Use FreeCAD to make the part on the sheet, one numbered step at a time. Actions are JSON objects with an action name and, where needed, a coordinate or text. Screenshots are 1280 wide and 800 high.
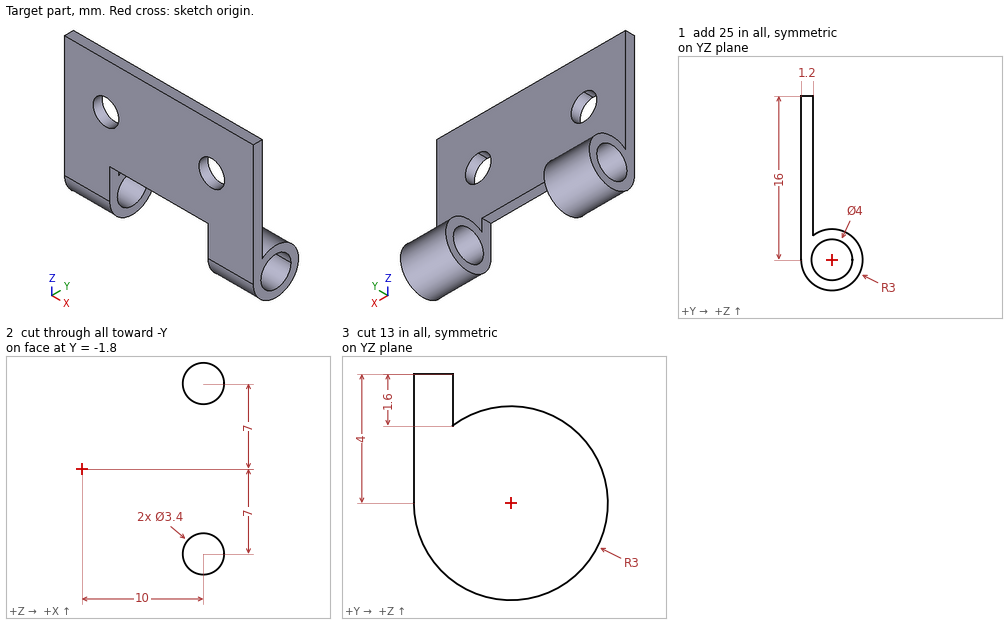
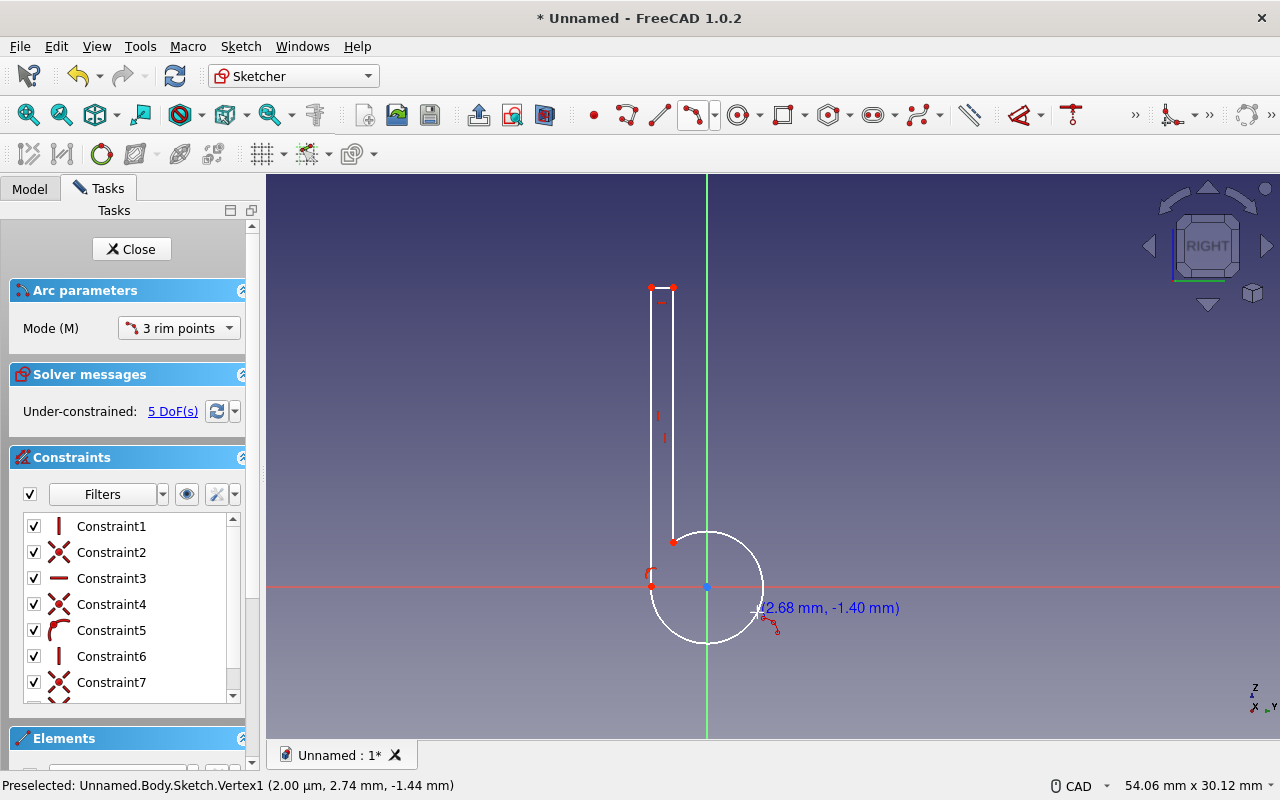
{"action": "key", "text": "g c"}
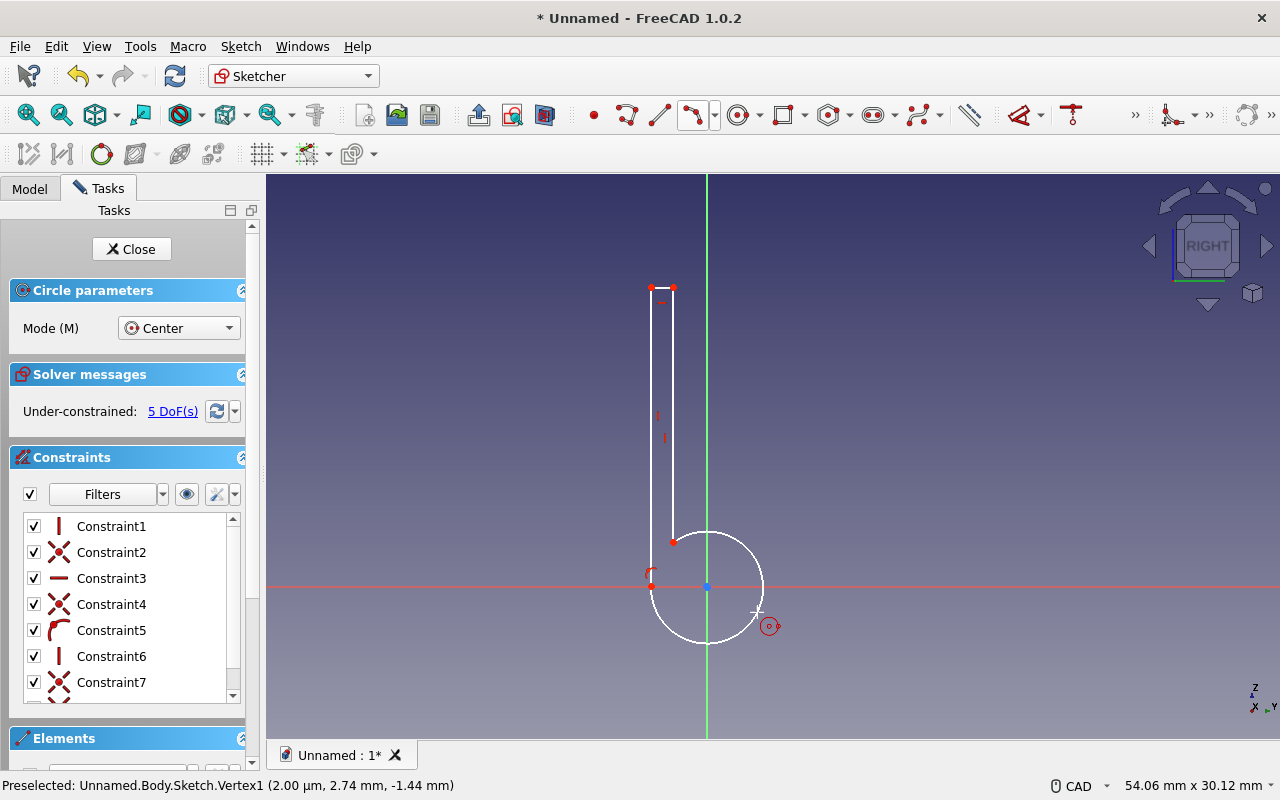
{"action": "left_click", "coordinate": [707, 587]}
{"action": "left_click", "coordinate": [733, 560]}
{"action": "key", "text": "Escape"}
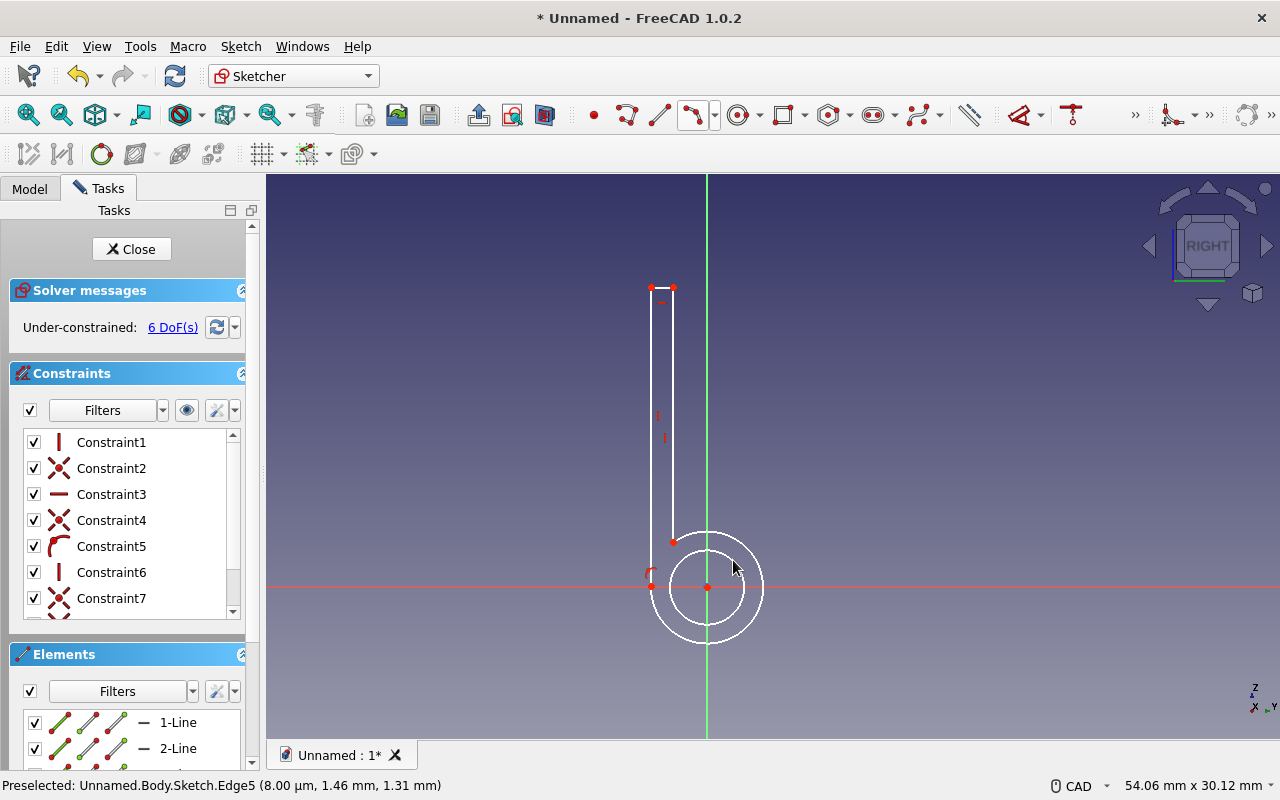
{"action": "left_click", "coordinate": [651, 378]}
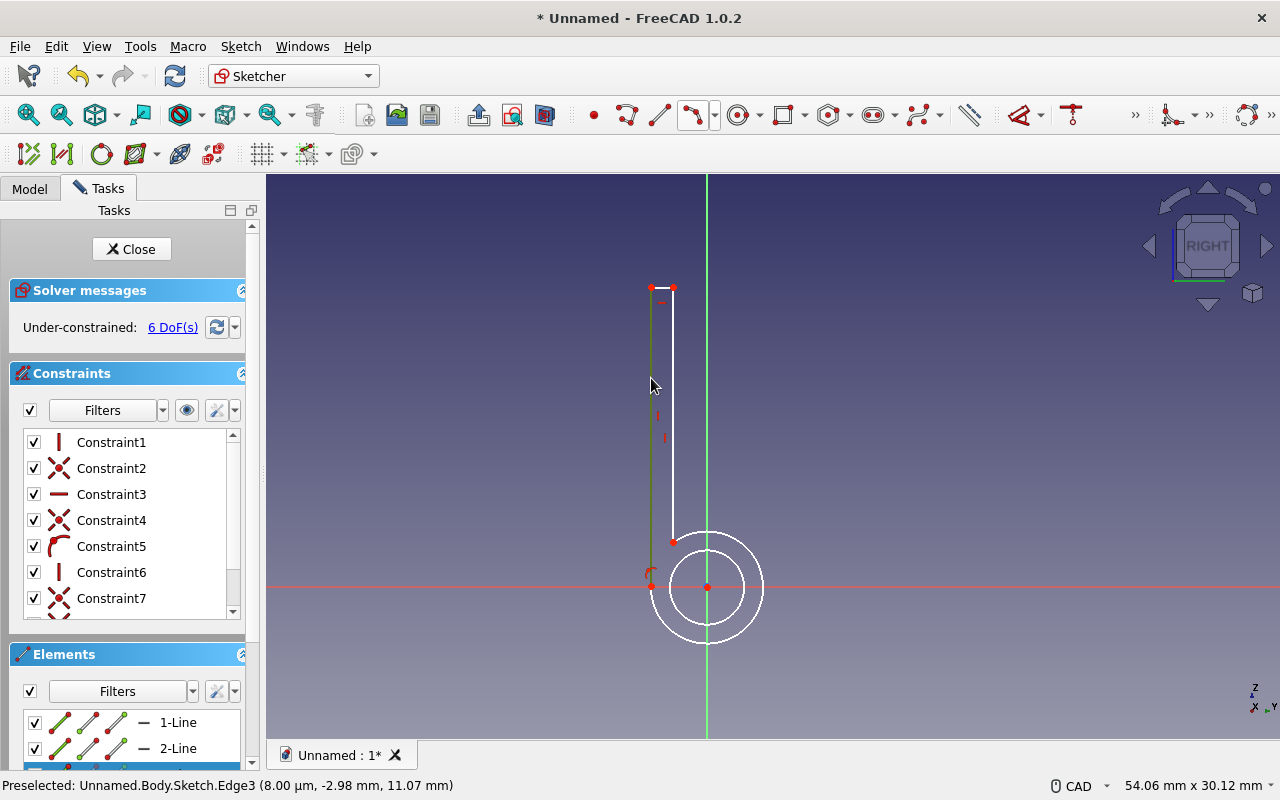
{"action": "left_click", "coordinate": [709, 644]}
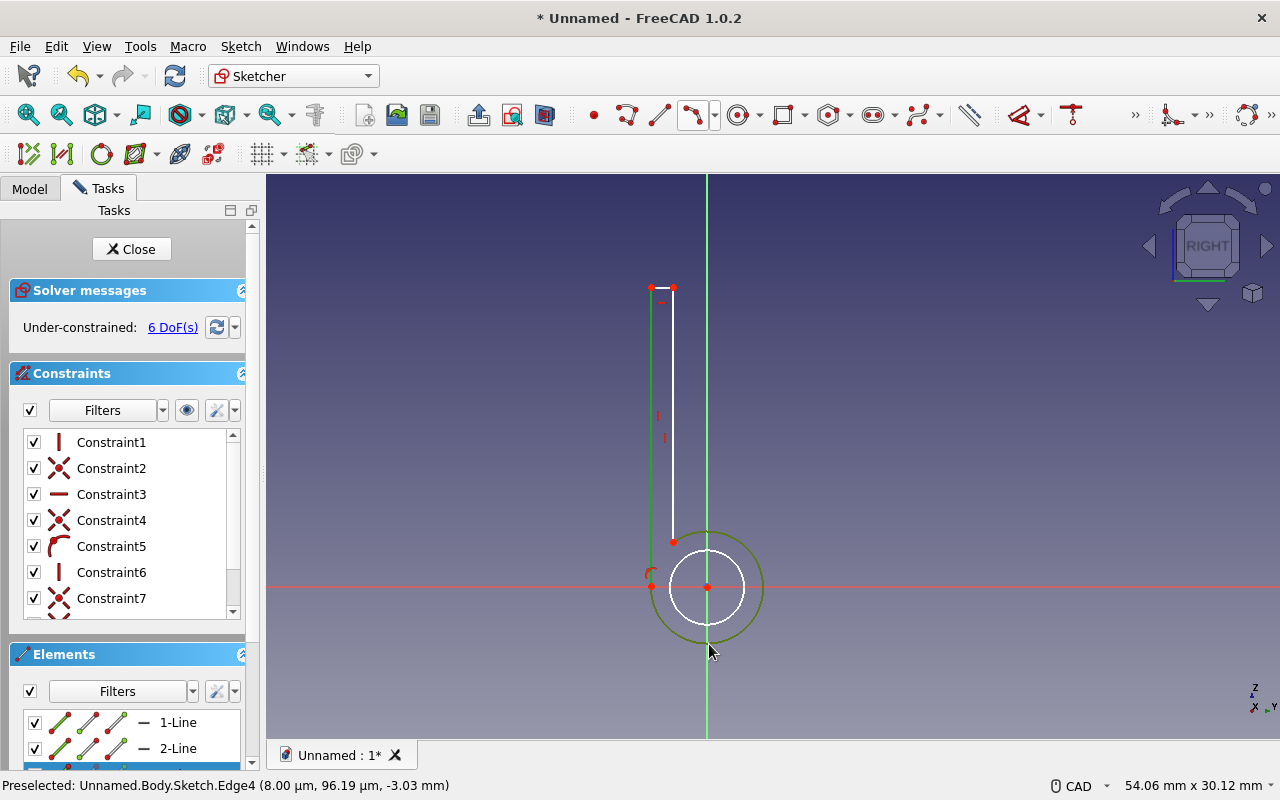
{"action": "key", "text": "t"}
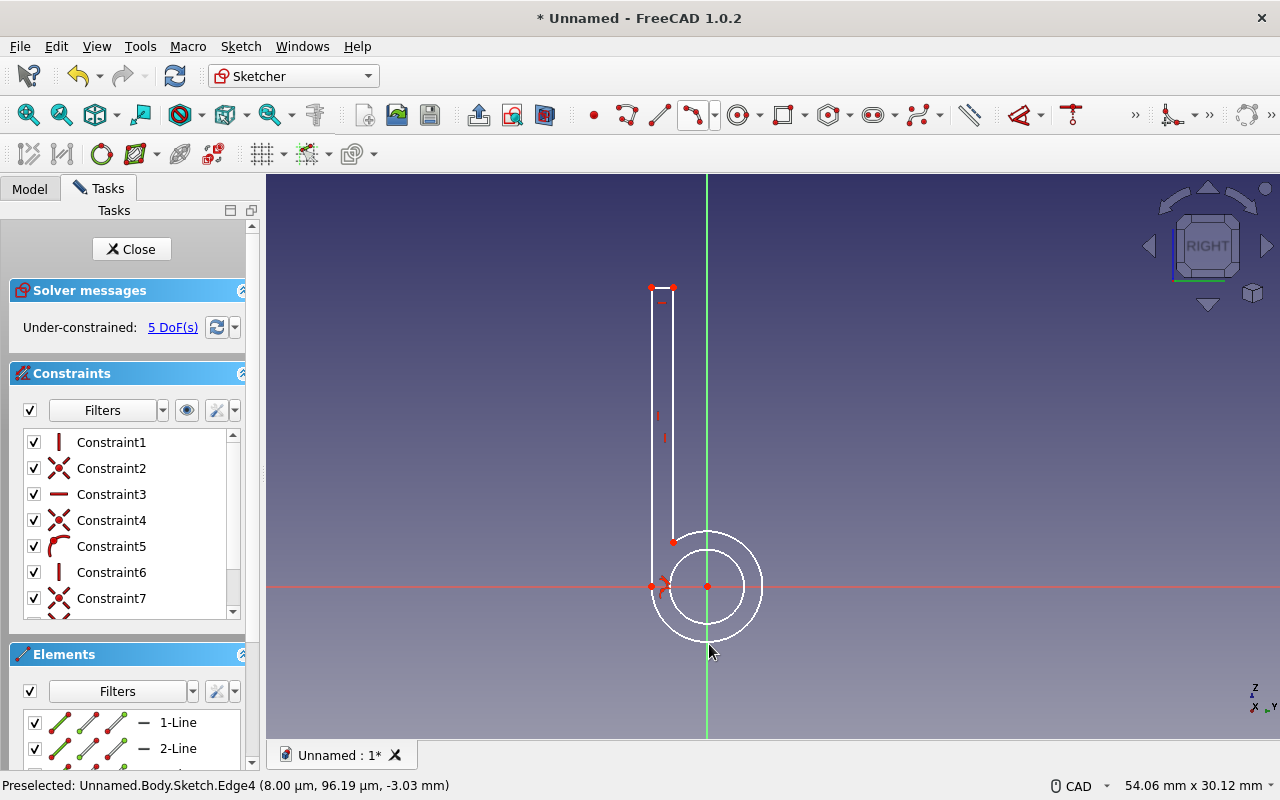
{"action": "left_click", "coordinate": [707, 587]}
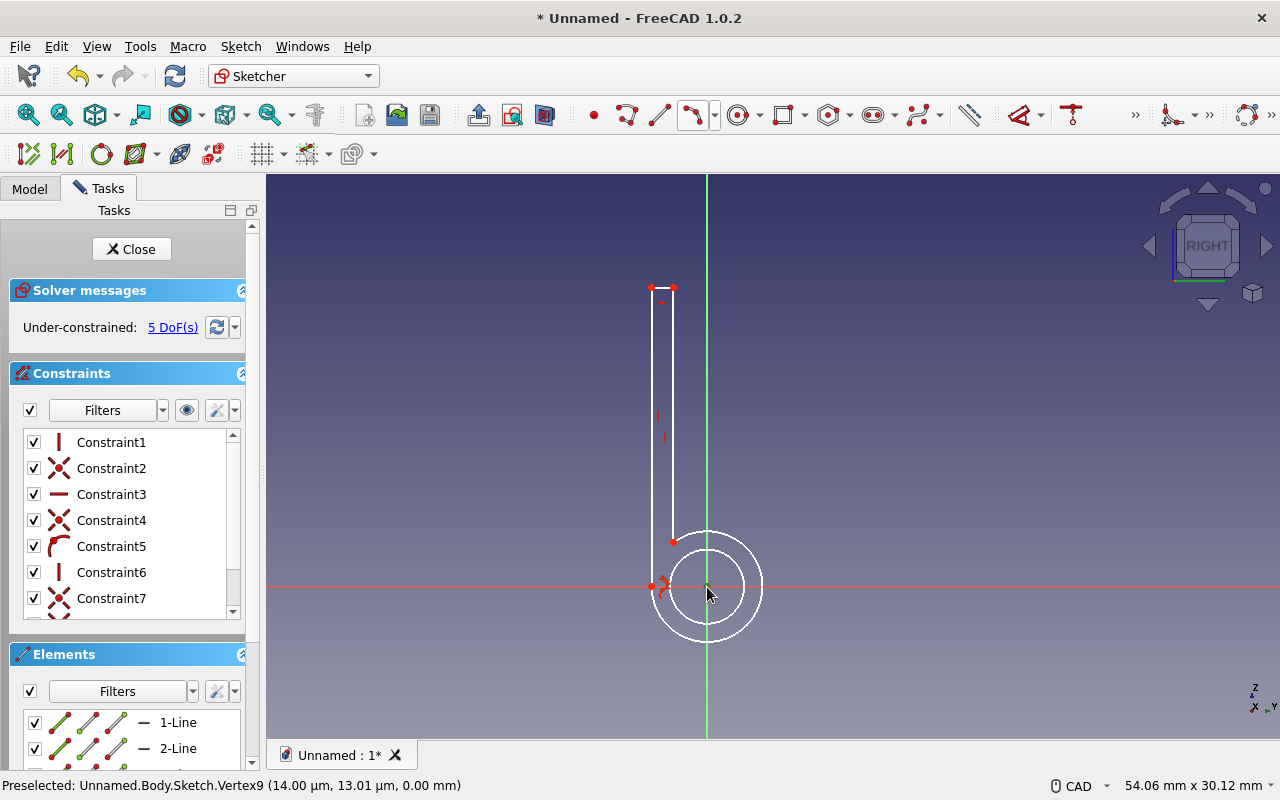
{"action": "left_click", "coordinate": [707, 675]}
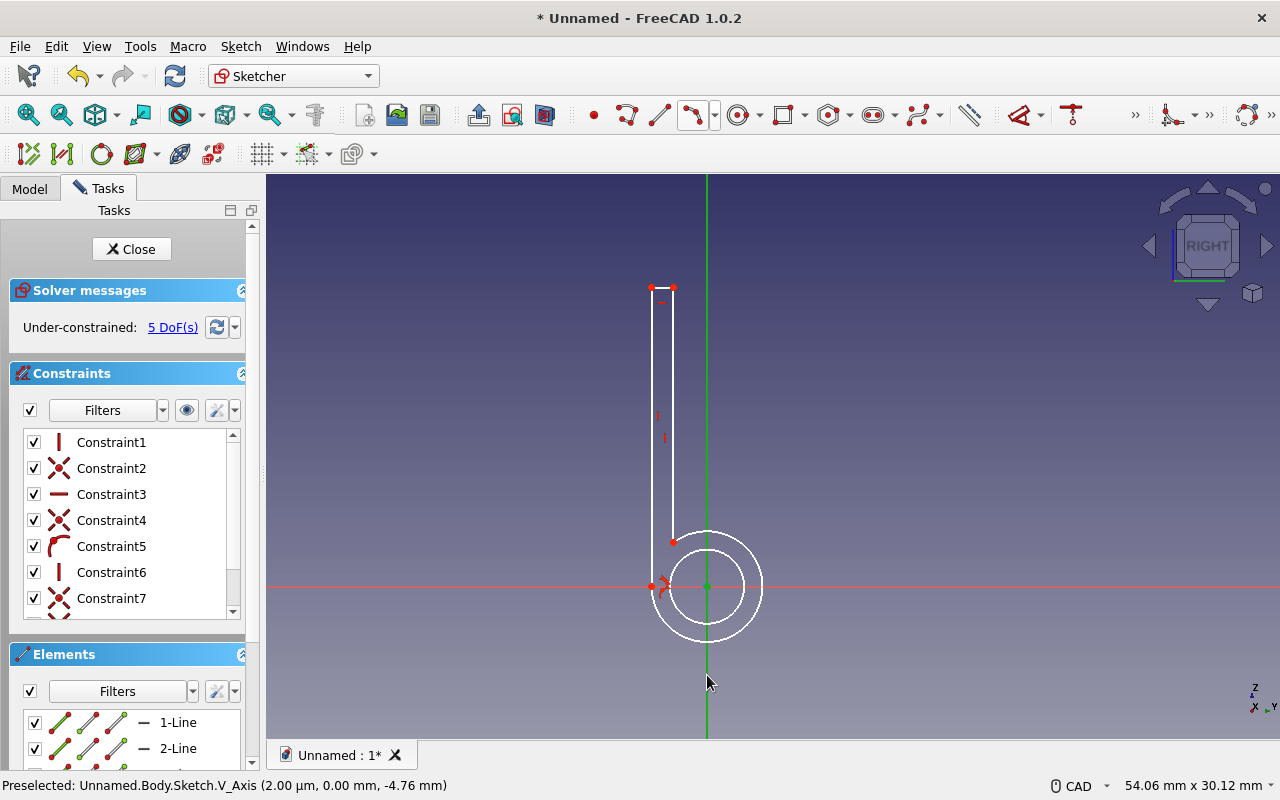
{"action": "key", "text": "c"}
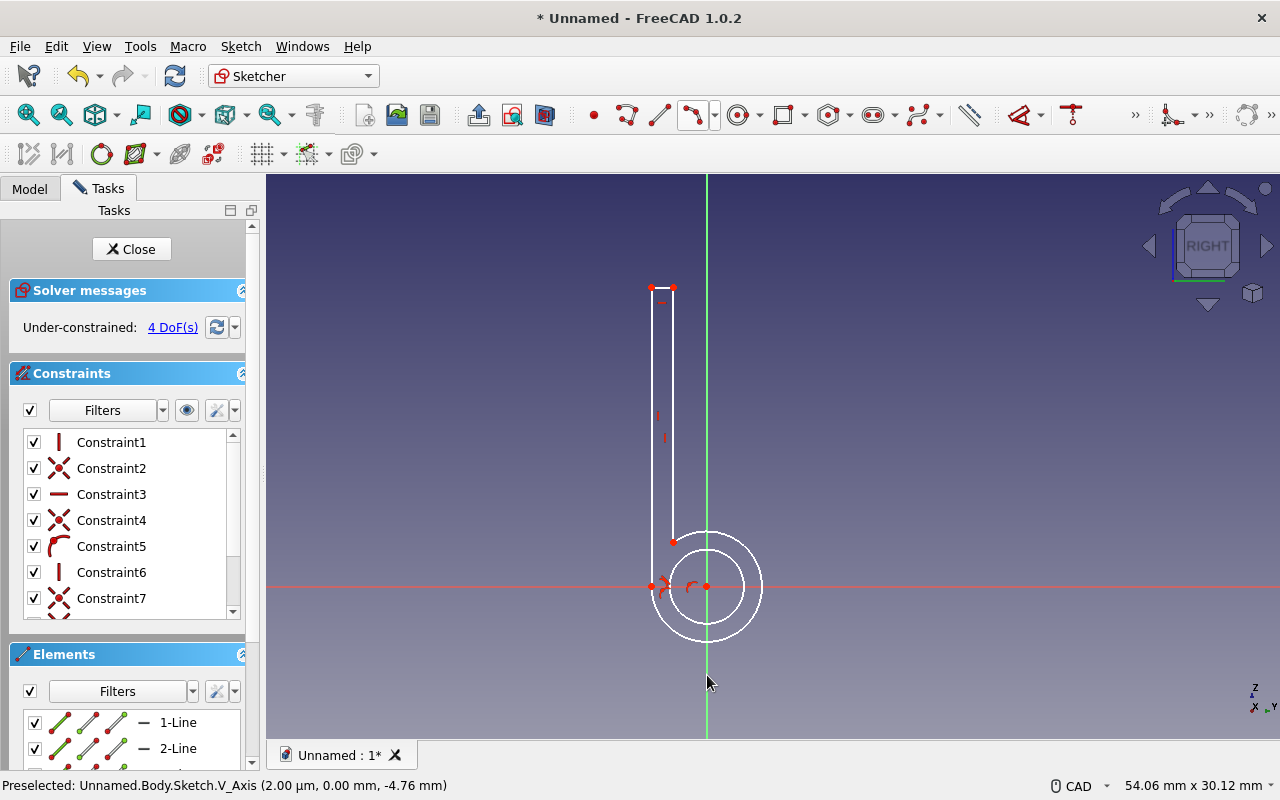
{"action": "left_click", "coordinate": [1018, 116]}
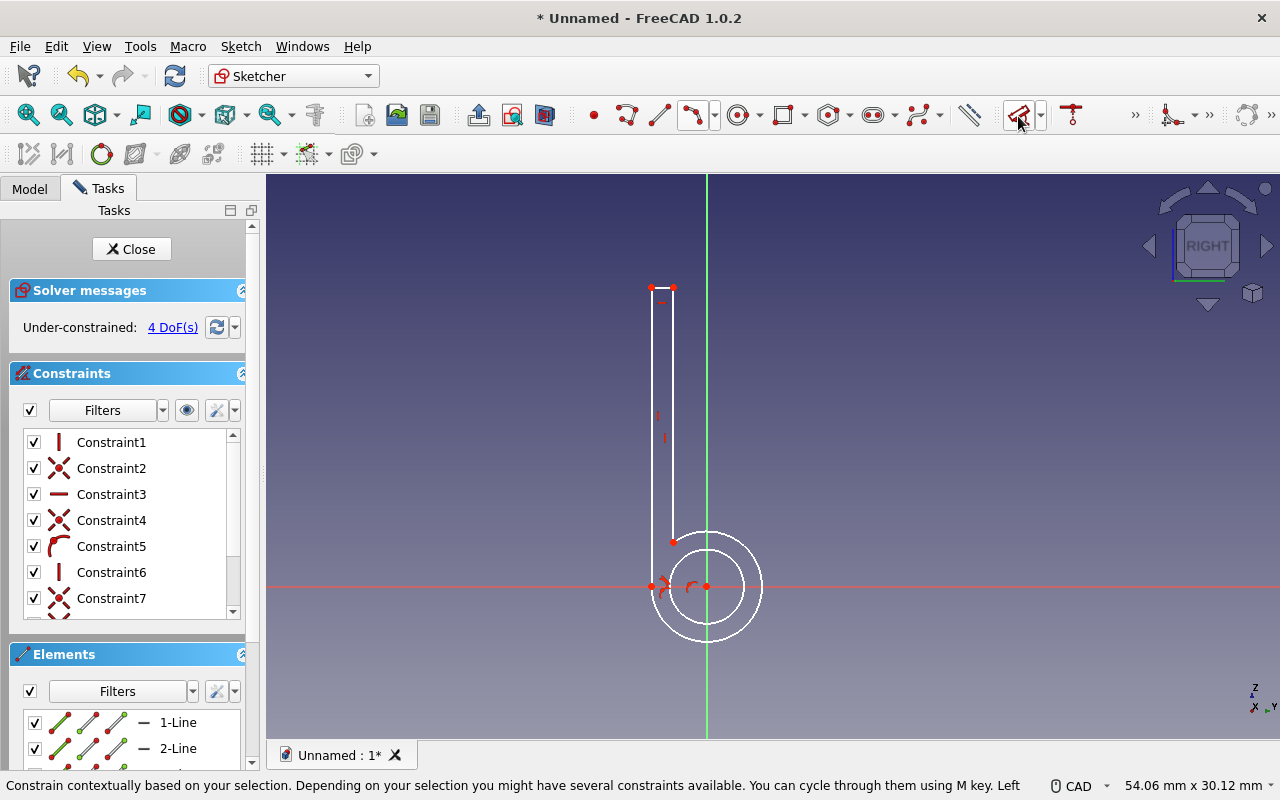
{"action": "left_click", "coordinate": [709, 642]}
{"action": "left_click", "coordinate": [668, 665]}